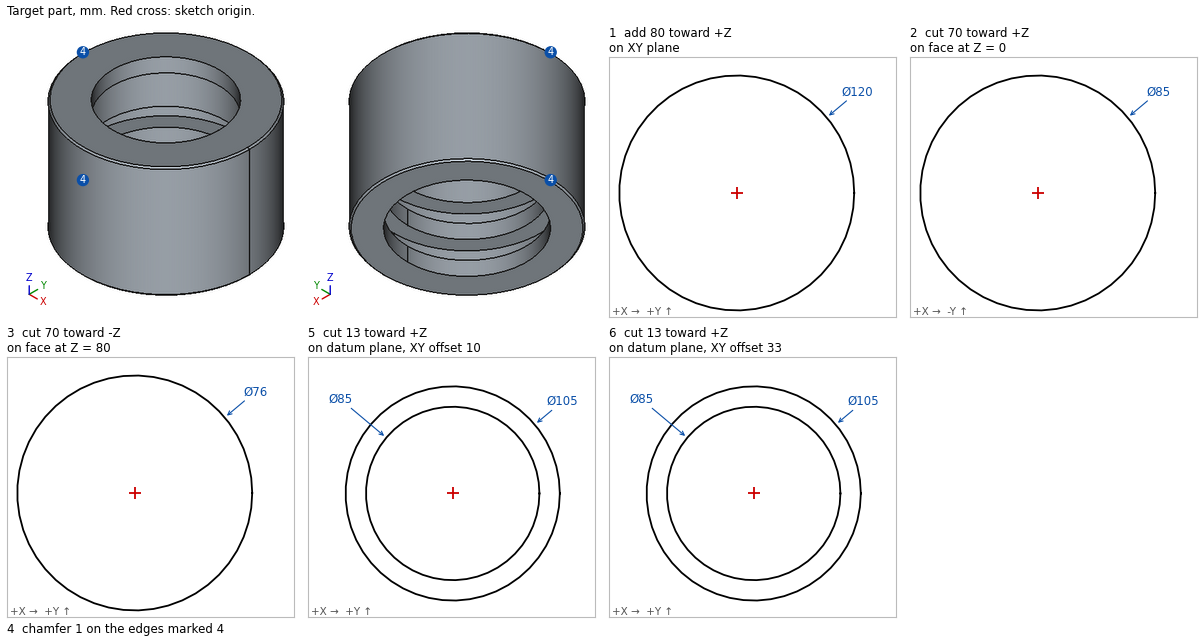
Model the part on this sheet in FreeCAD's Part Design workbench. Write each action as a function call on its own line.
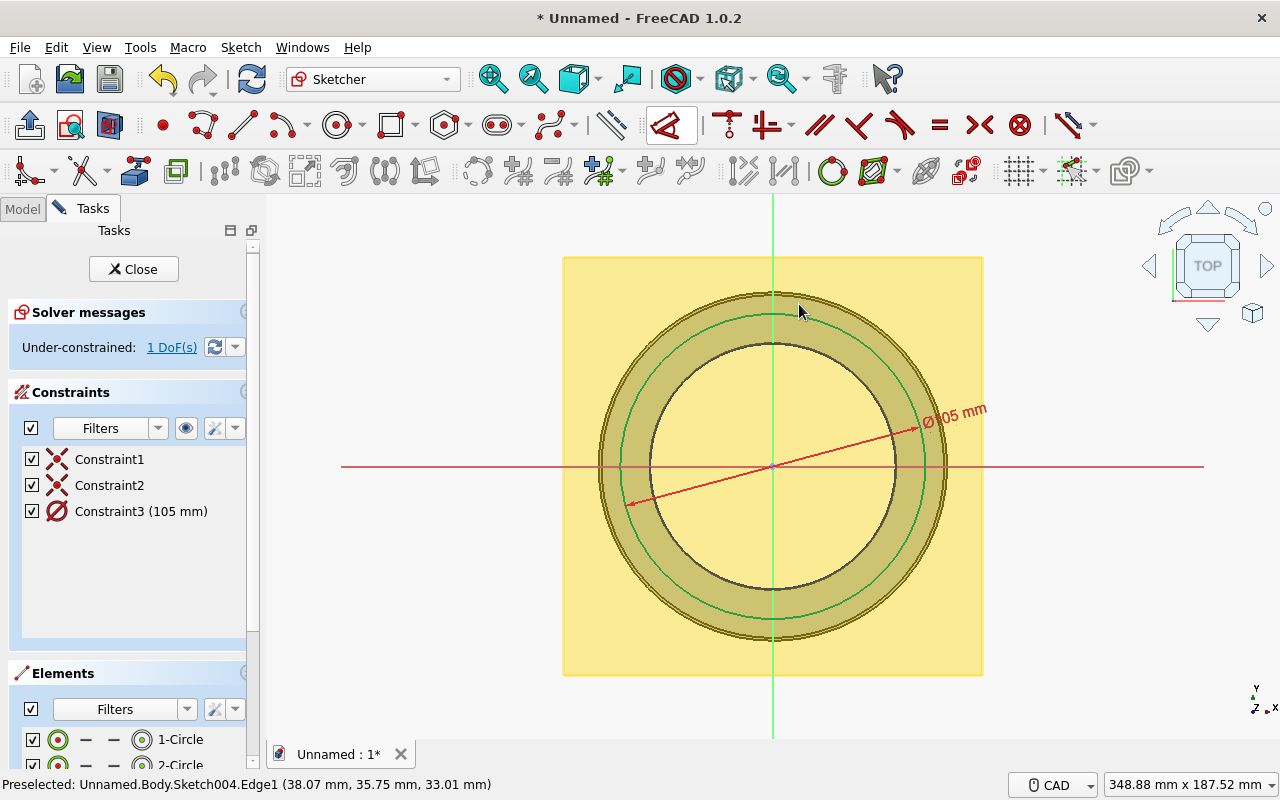
click(859, 379)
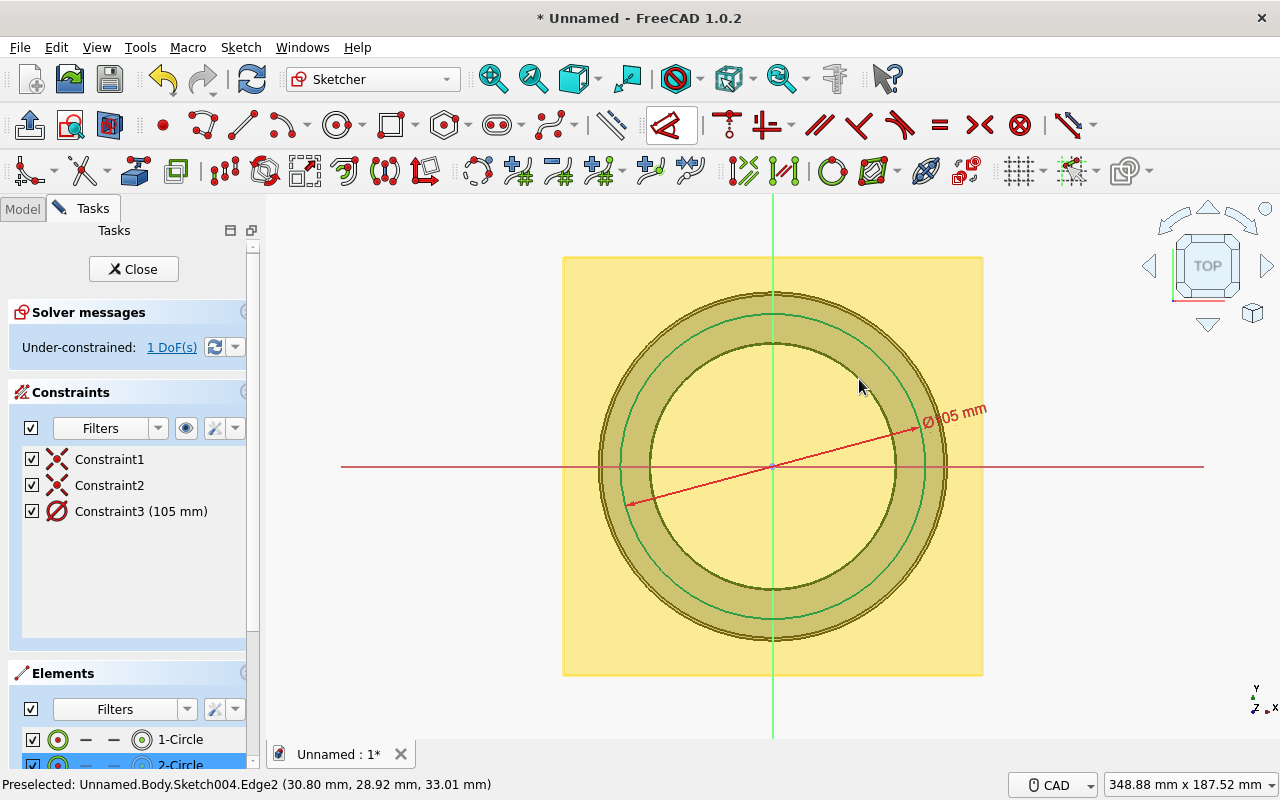
click(692, 126)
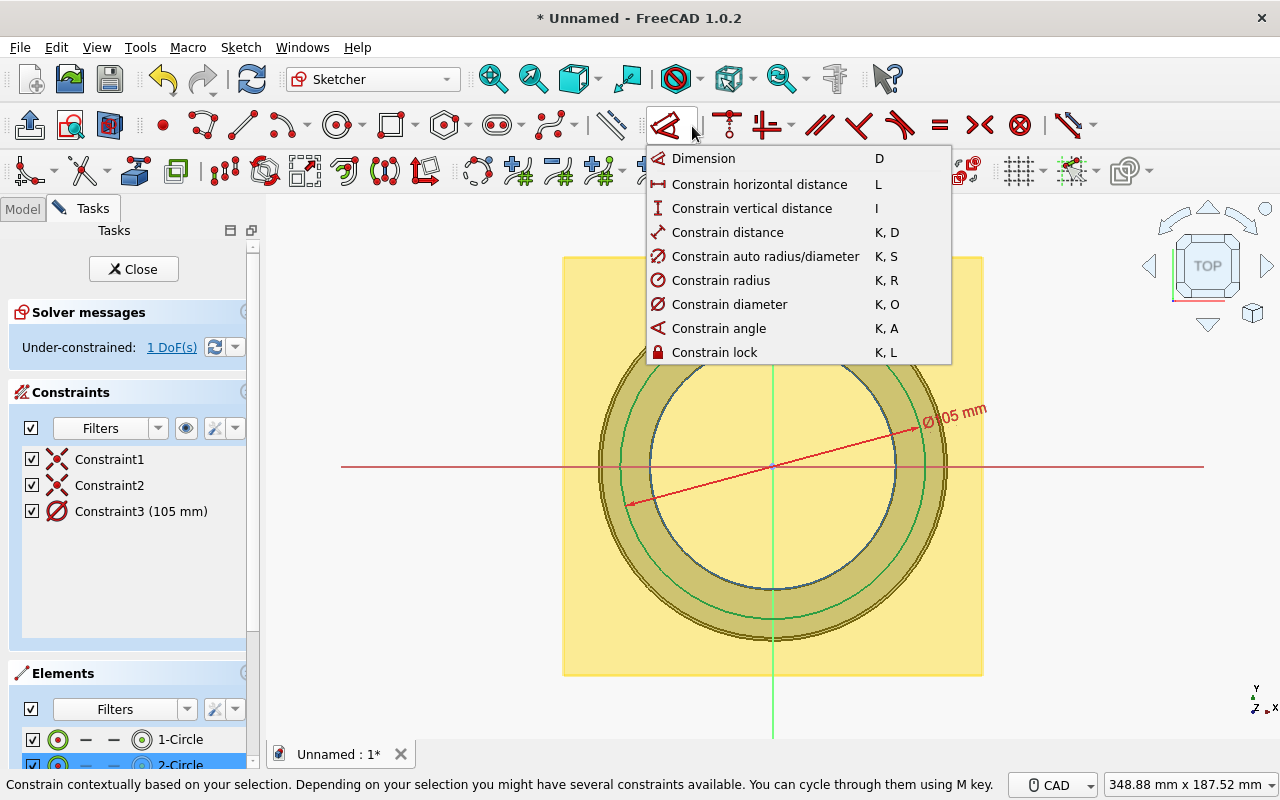
click(799, 304)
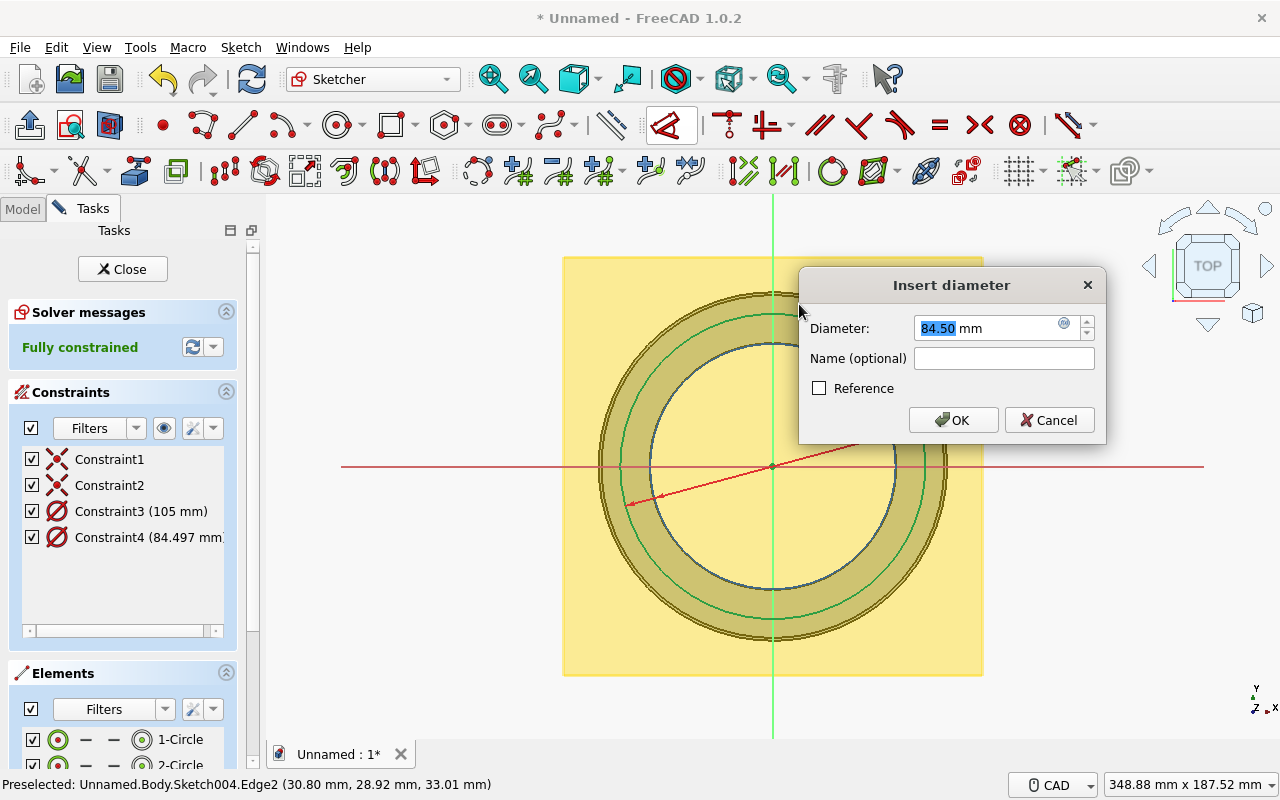
text(85)
key(Return)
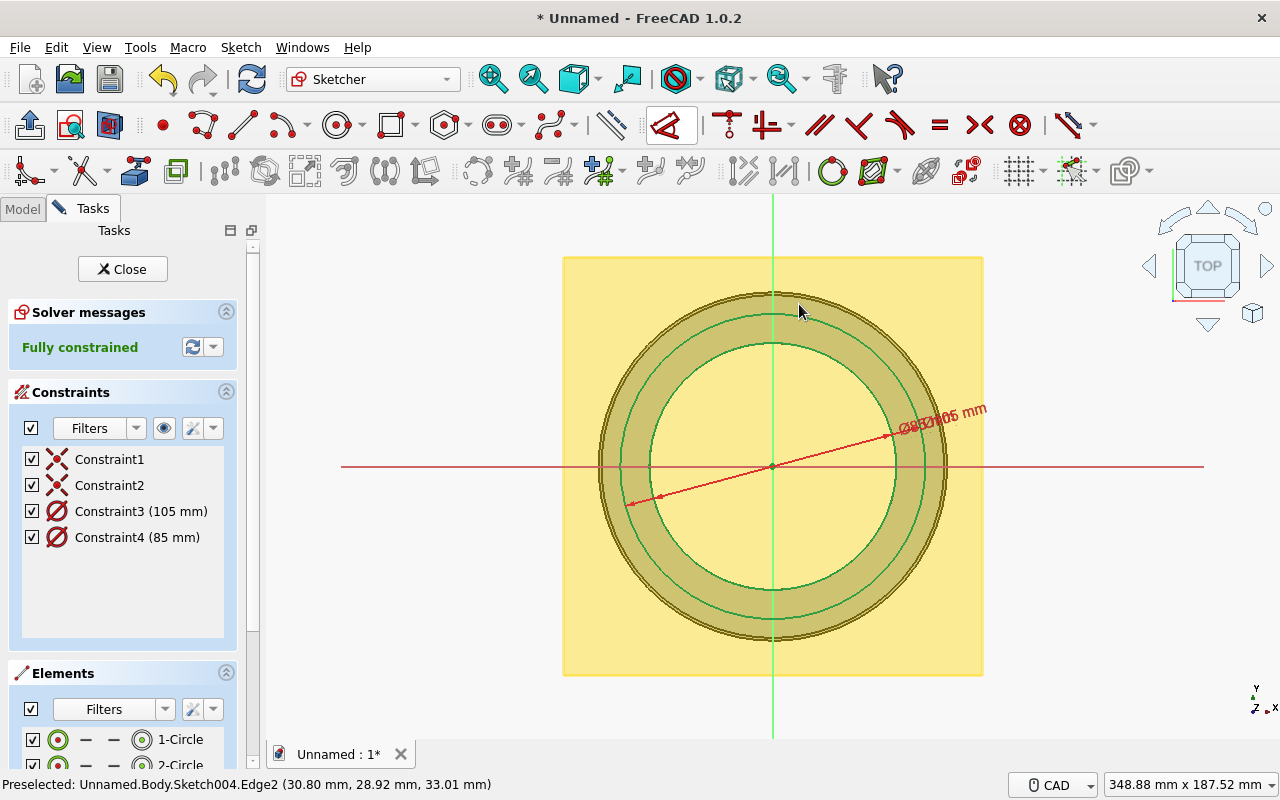
click(123, 269)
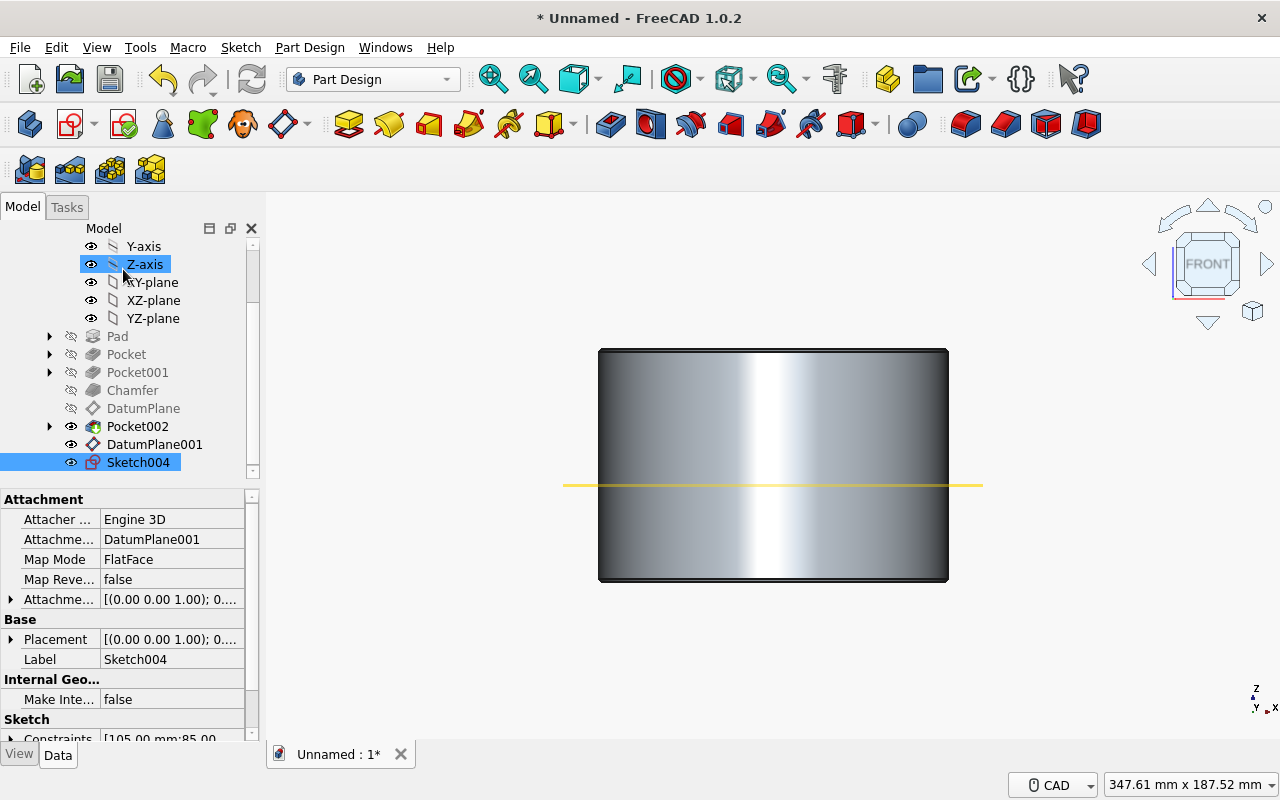
click(612, 124)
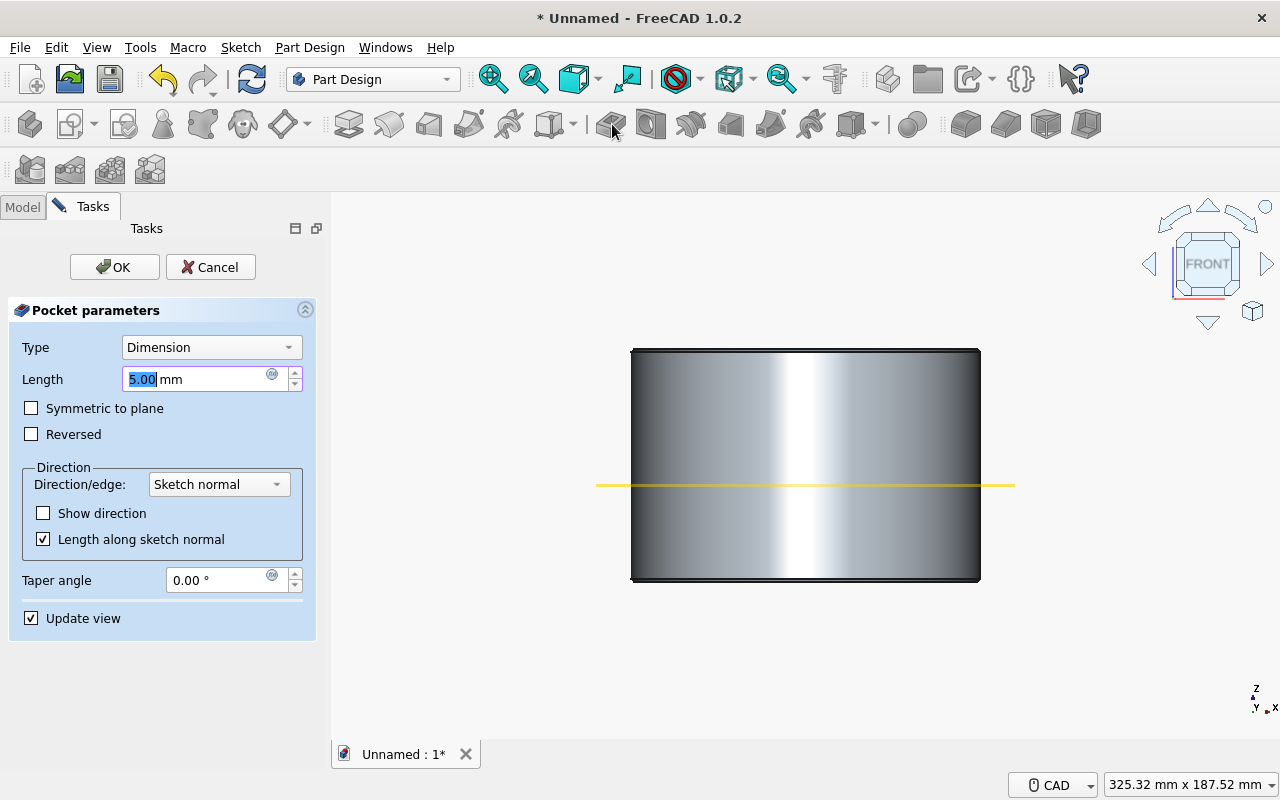
text(13)
key(Tab)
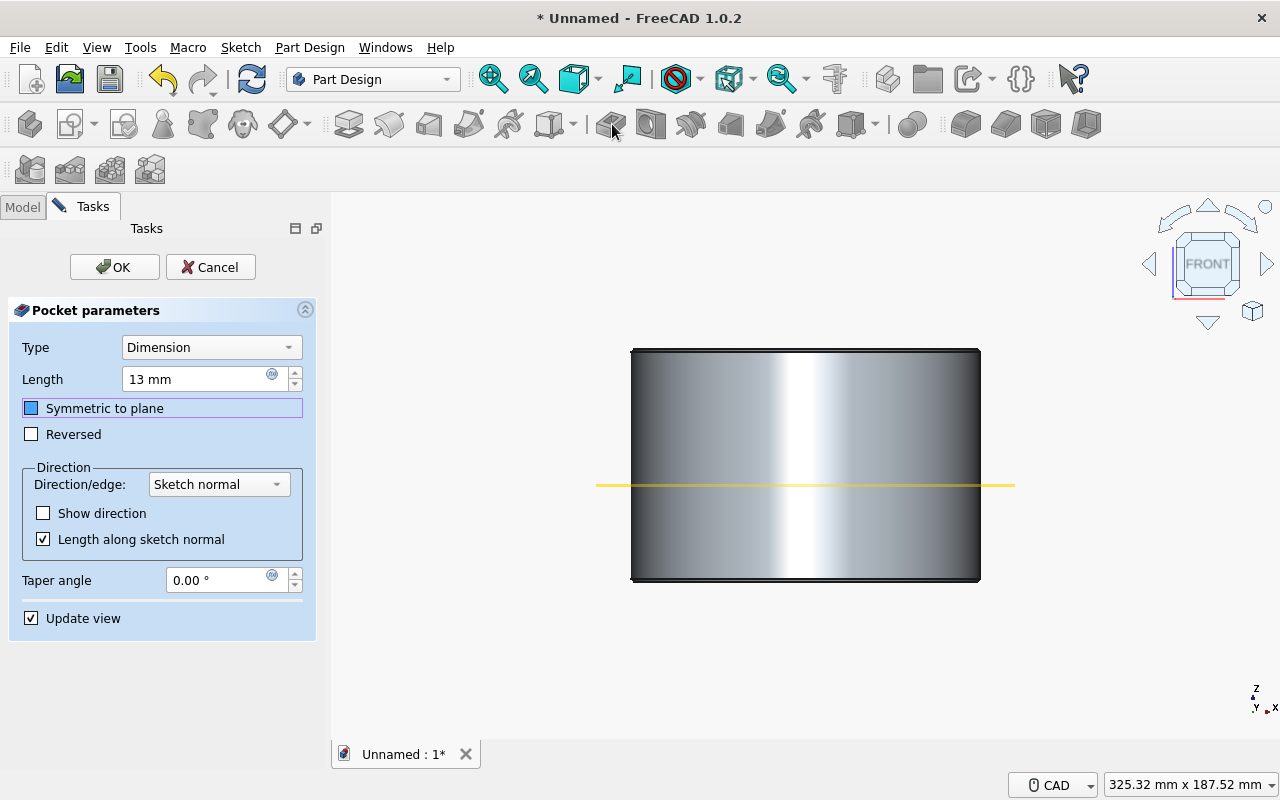
click(30, 434)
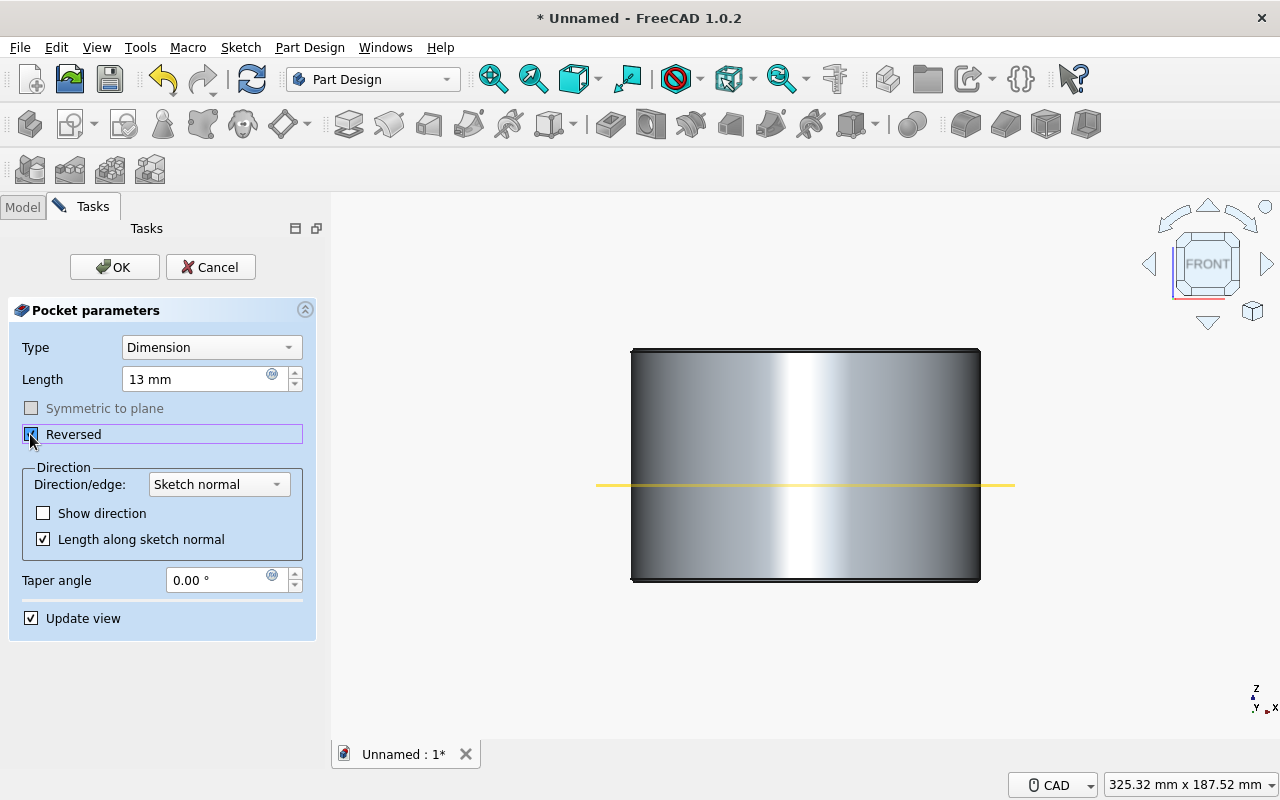
click(115, 267)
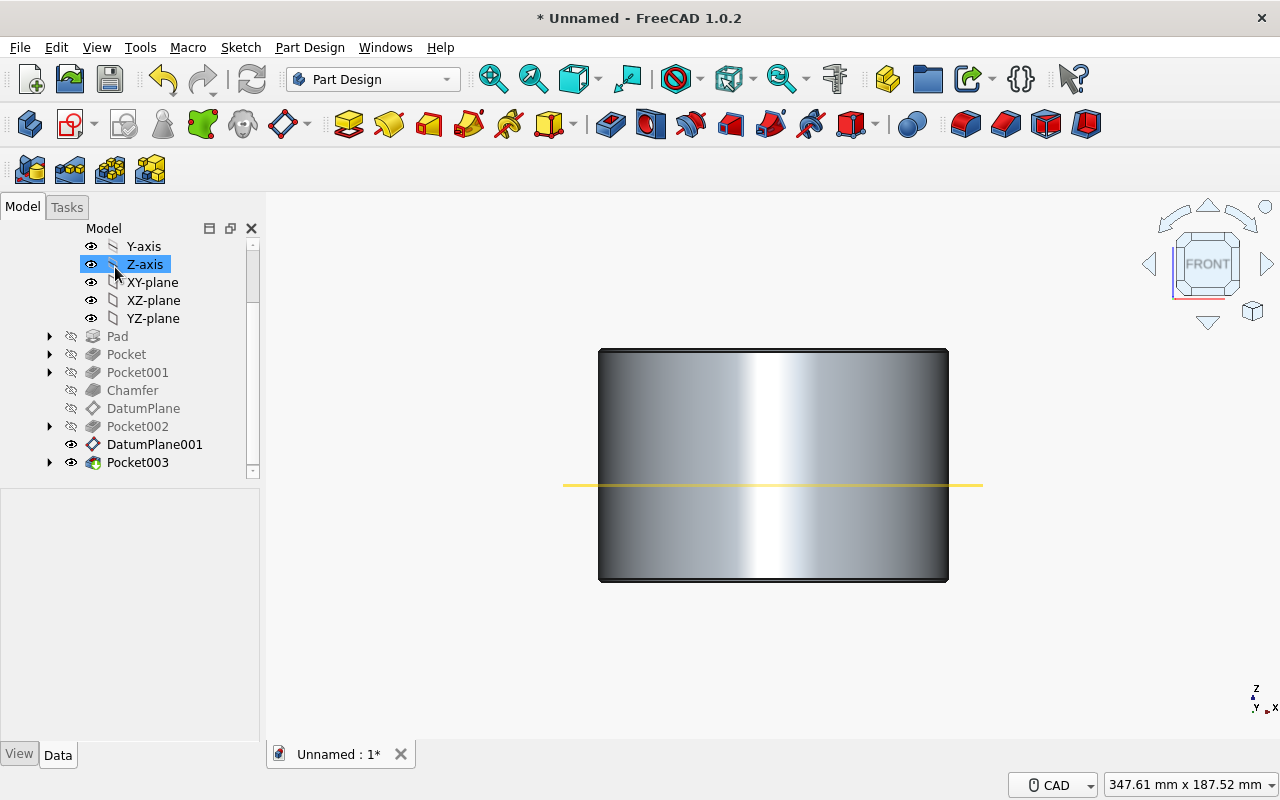
click(116, 444)
key(space)